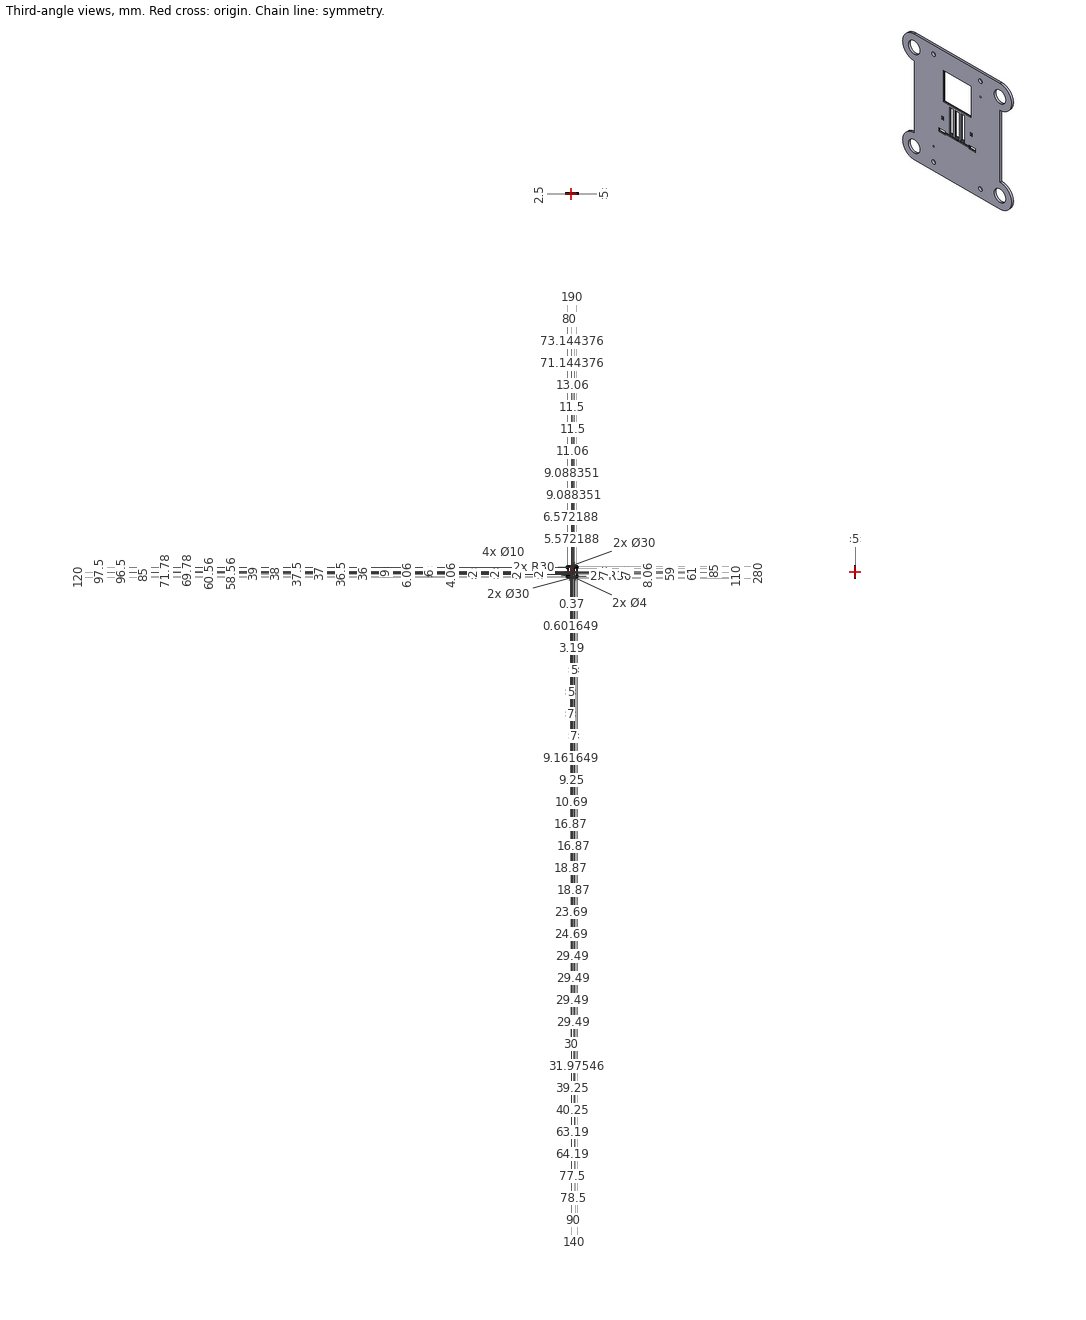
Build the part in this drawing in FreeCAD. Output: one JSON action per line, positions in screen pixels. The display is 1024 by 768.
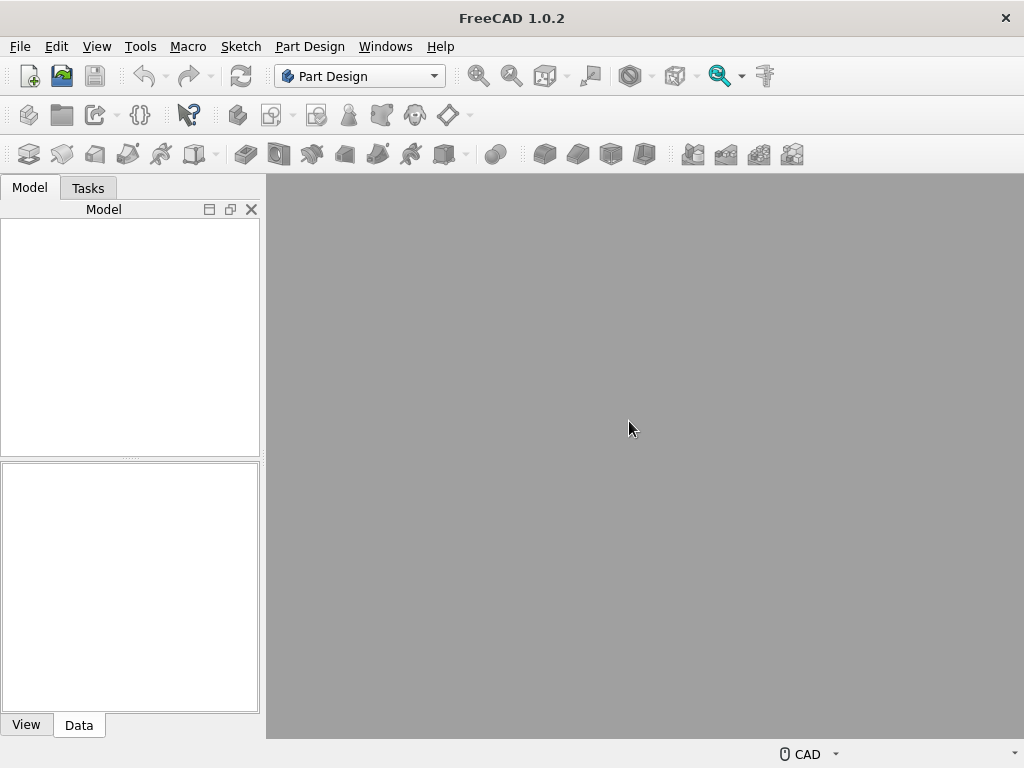
{"action": "left_click", "coordinate": [29, 76]}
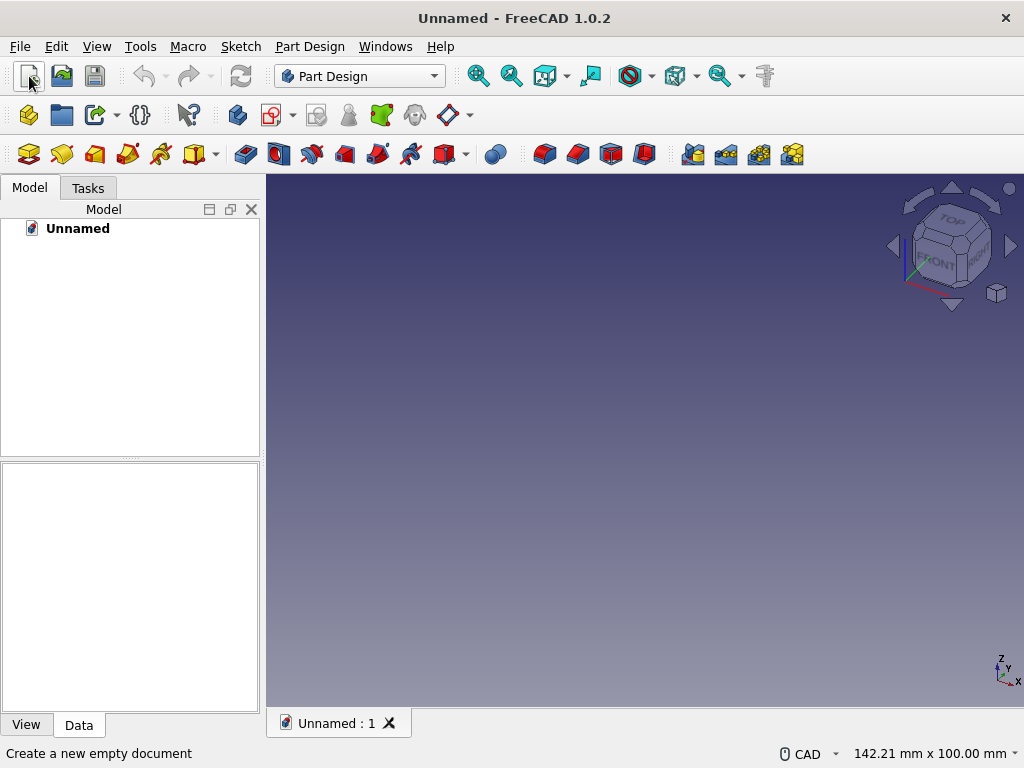
{"action": "left_click", "coordinate": [270, 116]}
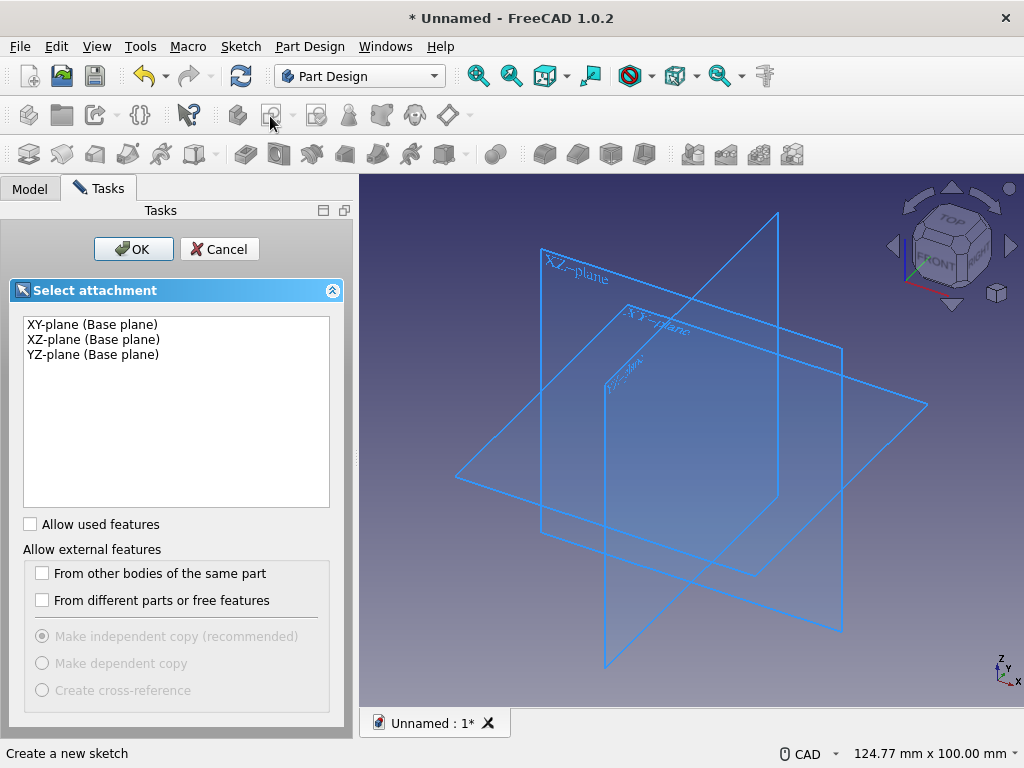
{"action": "left_click", "coordinate": [84, 340]}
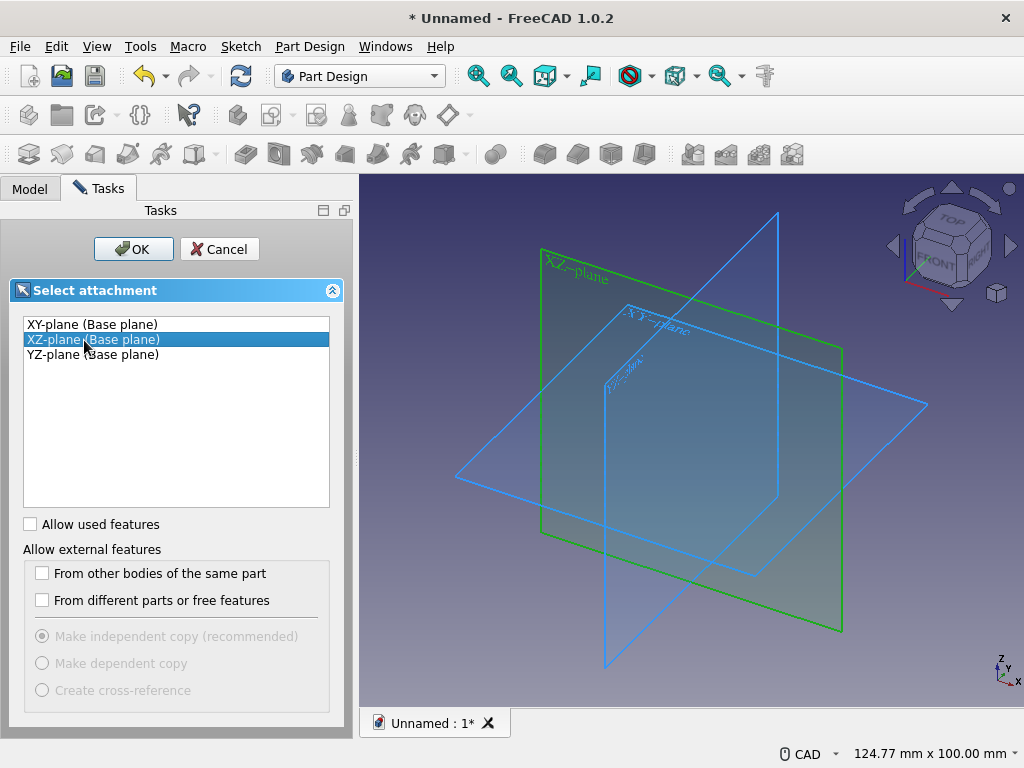
{"action": "left_click", "coordinate": [134, 249]}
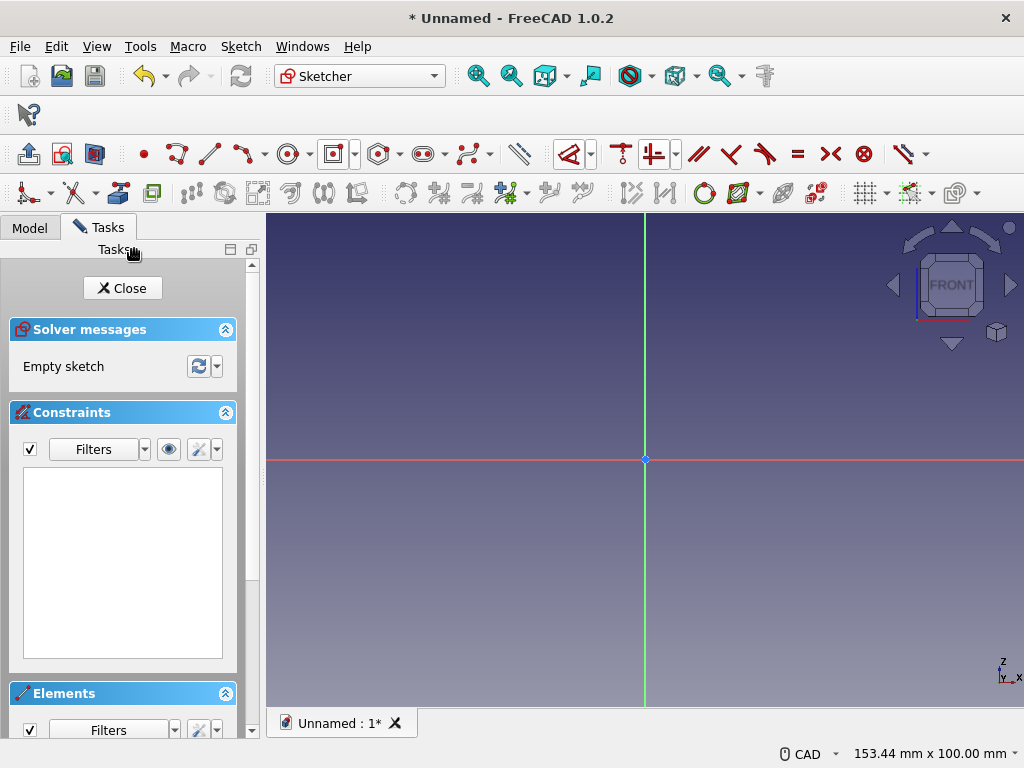
{"action": "scroll", "coordinate": [554, 460], "scroll_direction": "down", "scroll_amount": 7}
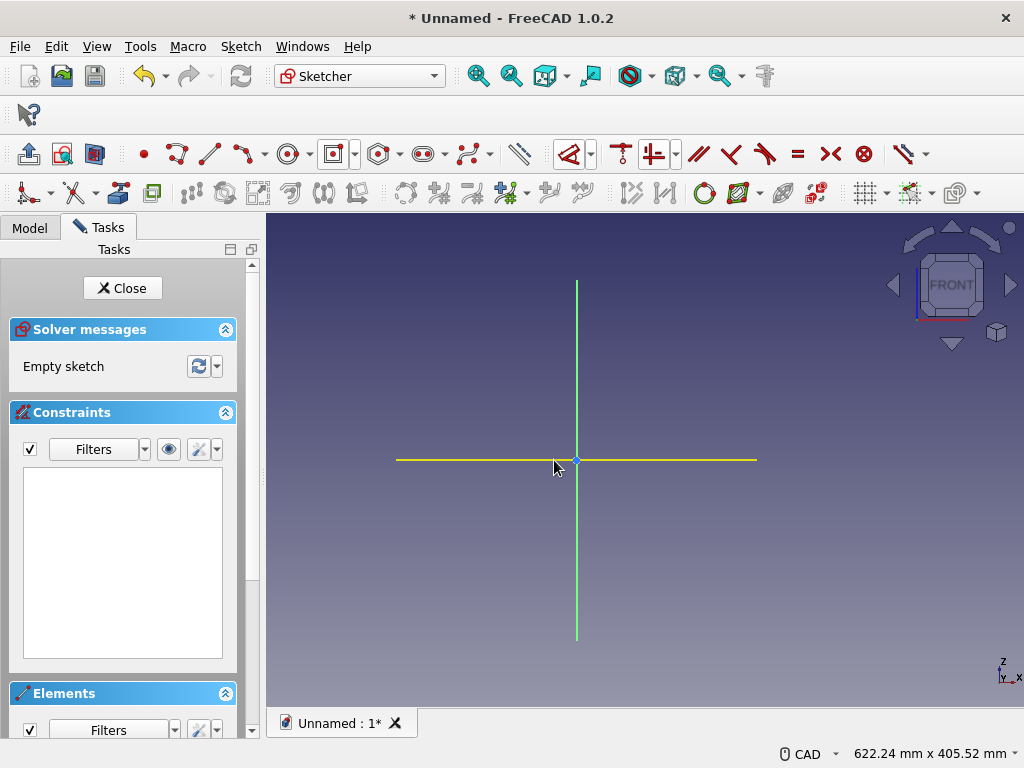
{"action": "left_click", "coordinate": [177, 154]}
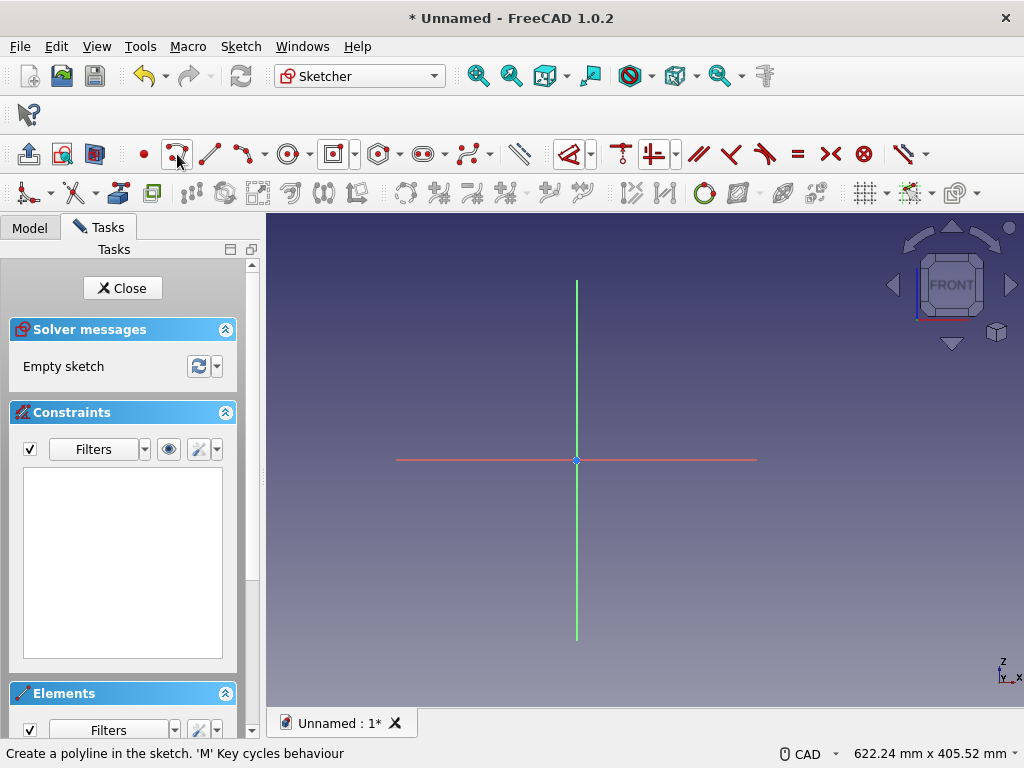
{"action": "left_click", "coordinate": [479, 290]}
{"action": "left_click", "coordinate": [711, 290]}
{"action": "left_click", "coordinate": [711, 631]}
{"action": "left_click", "coordinate": [479, 631]}
{"action": "right_click", "coordinate": [479, 631]}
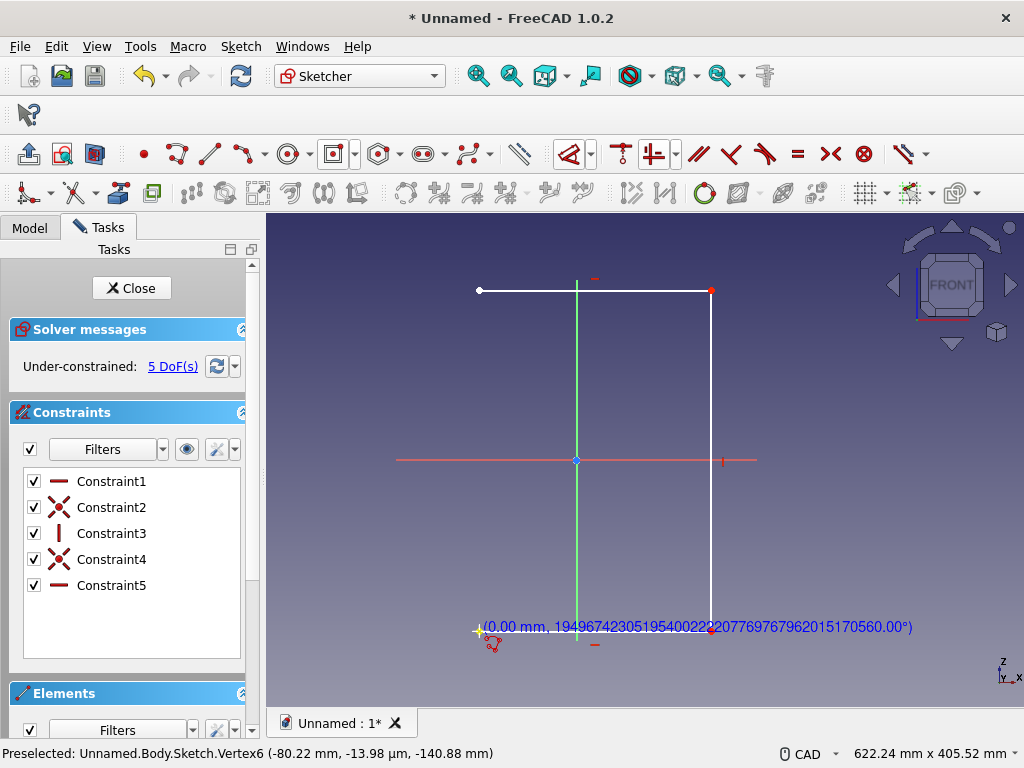
{"action": "key", "text": "g l"}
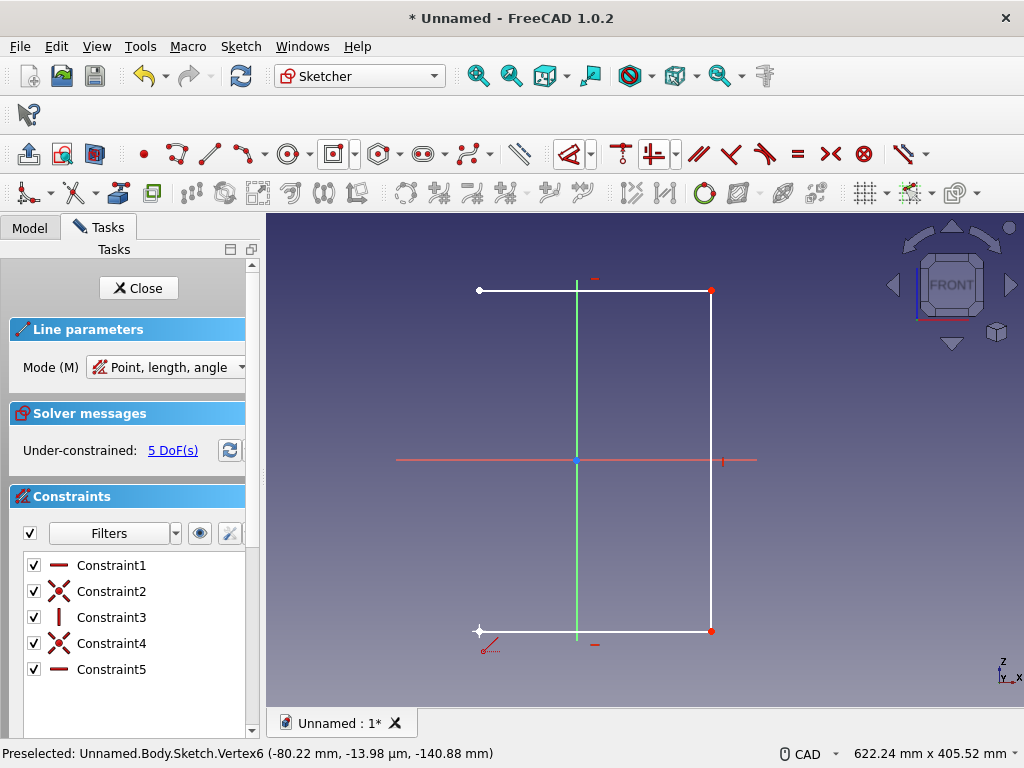
{"action": "left_click", "coordinate": [479, 558]}
{"action": "left_click", "coordinate": [479, 363]}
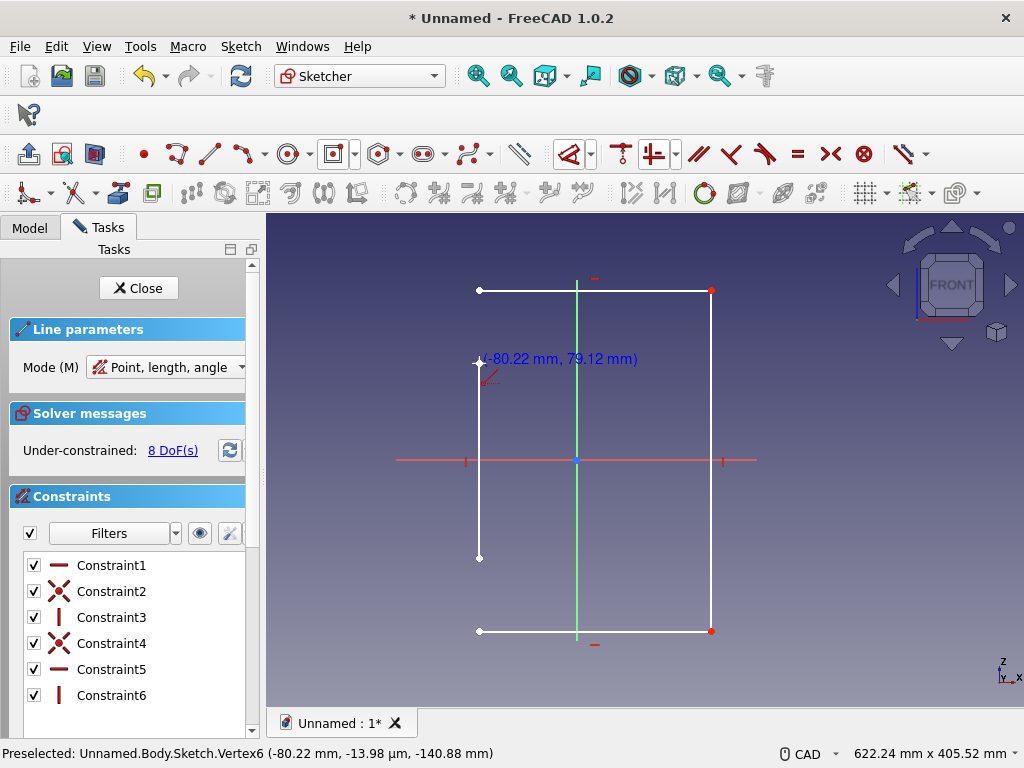
{"action": "left_click", "coordinate": [242, 154]}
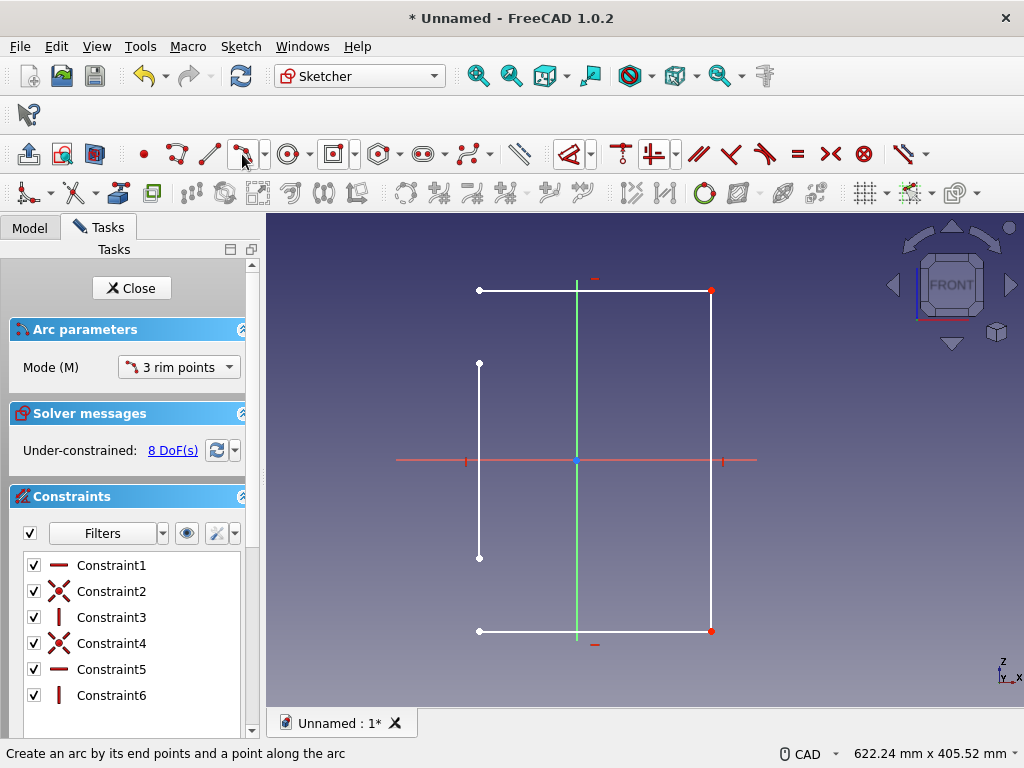
{"action": "left_click", "coordinate": [479, 632]}
{"action": "left_click", "coordinate": [479, 559]}
{"action": "left_click", "coordinate": [443, 594]}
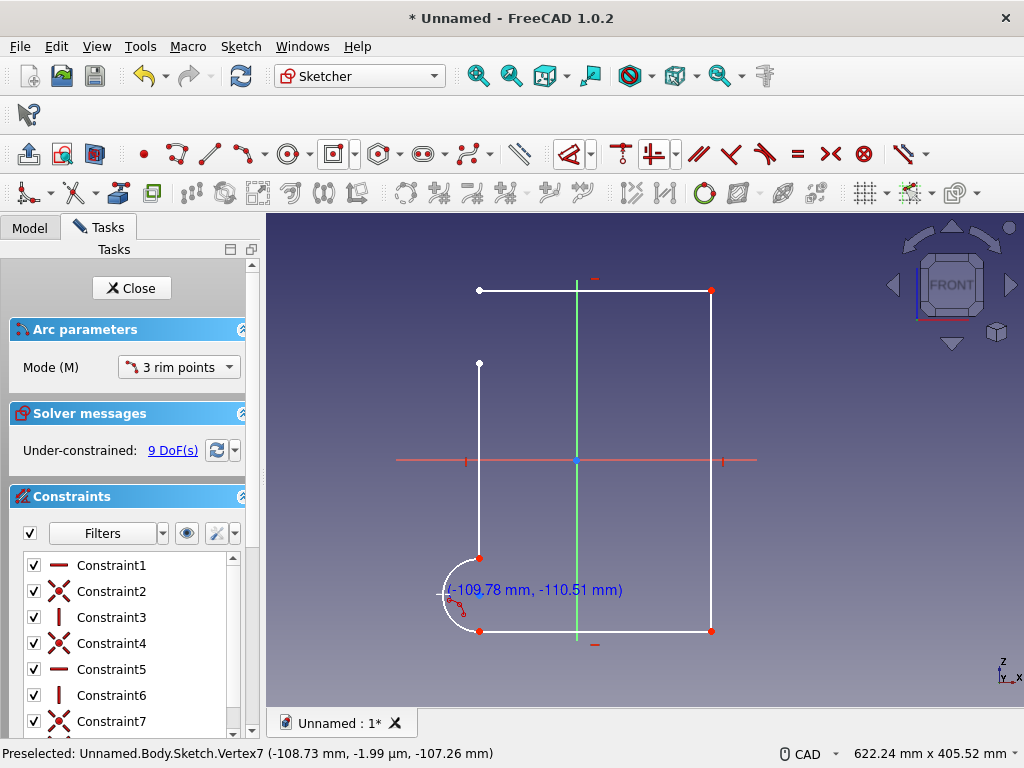
{"action": "left_click", "coordinate": [479, 364]}
{"action": "left_click", "coordinate": [479, 291]}
{"action": "left_click", "coordinate": [443, 326]}